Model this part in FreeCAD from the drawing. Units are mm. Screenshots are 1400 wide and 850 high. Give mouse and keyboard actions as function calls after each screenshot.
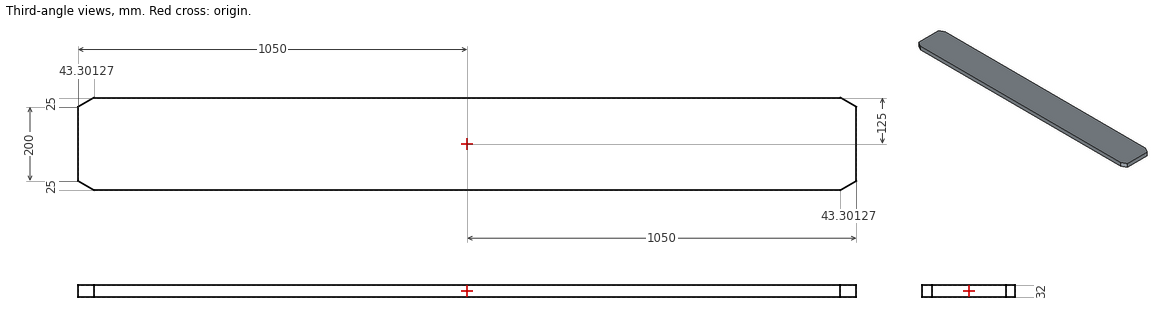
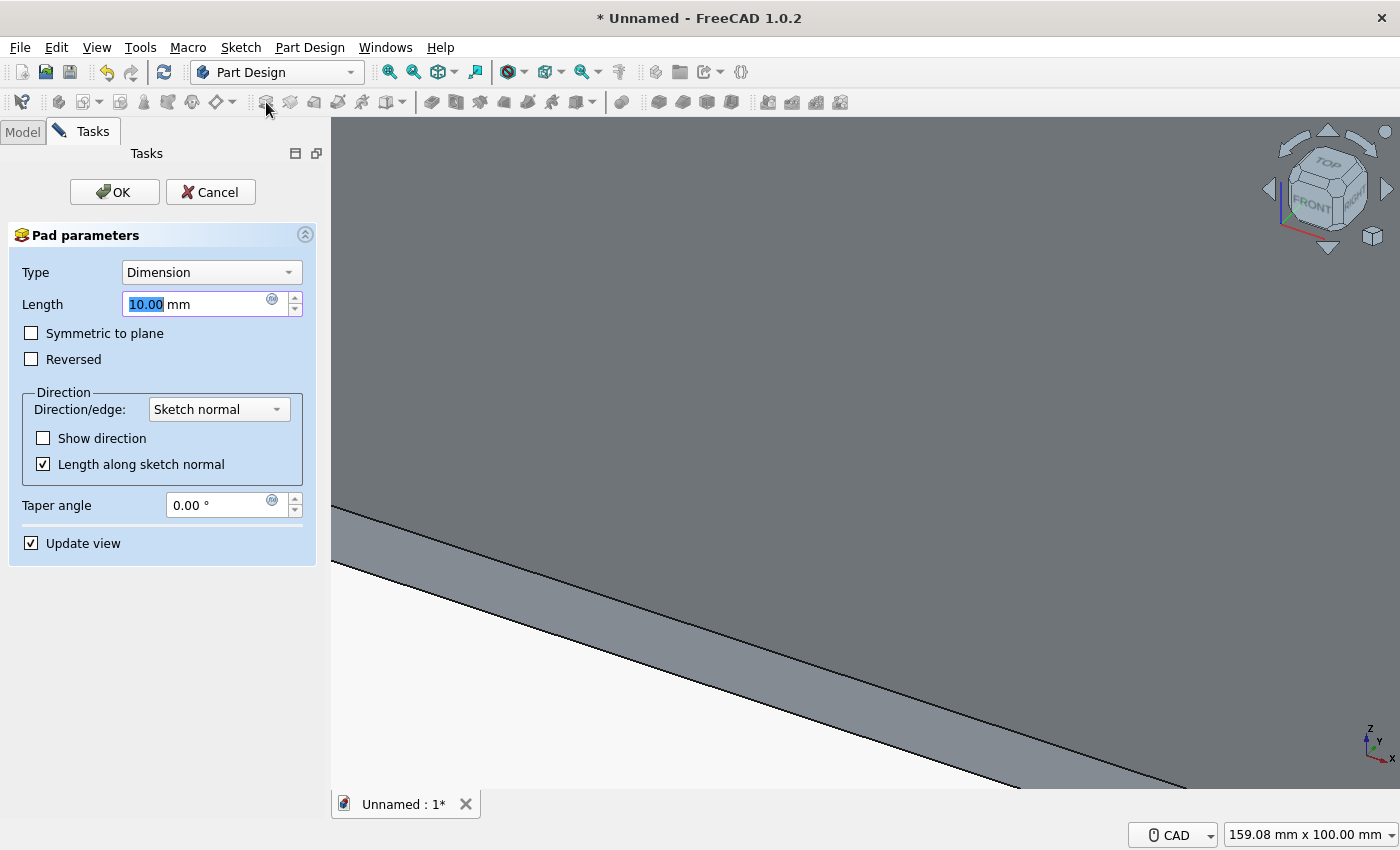
text(32)
key(Tab)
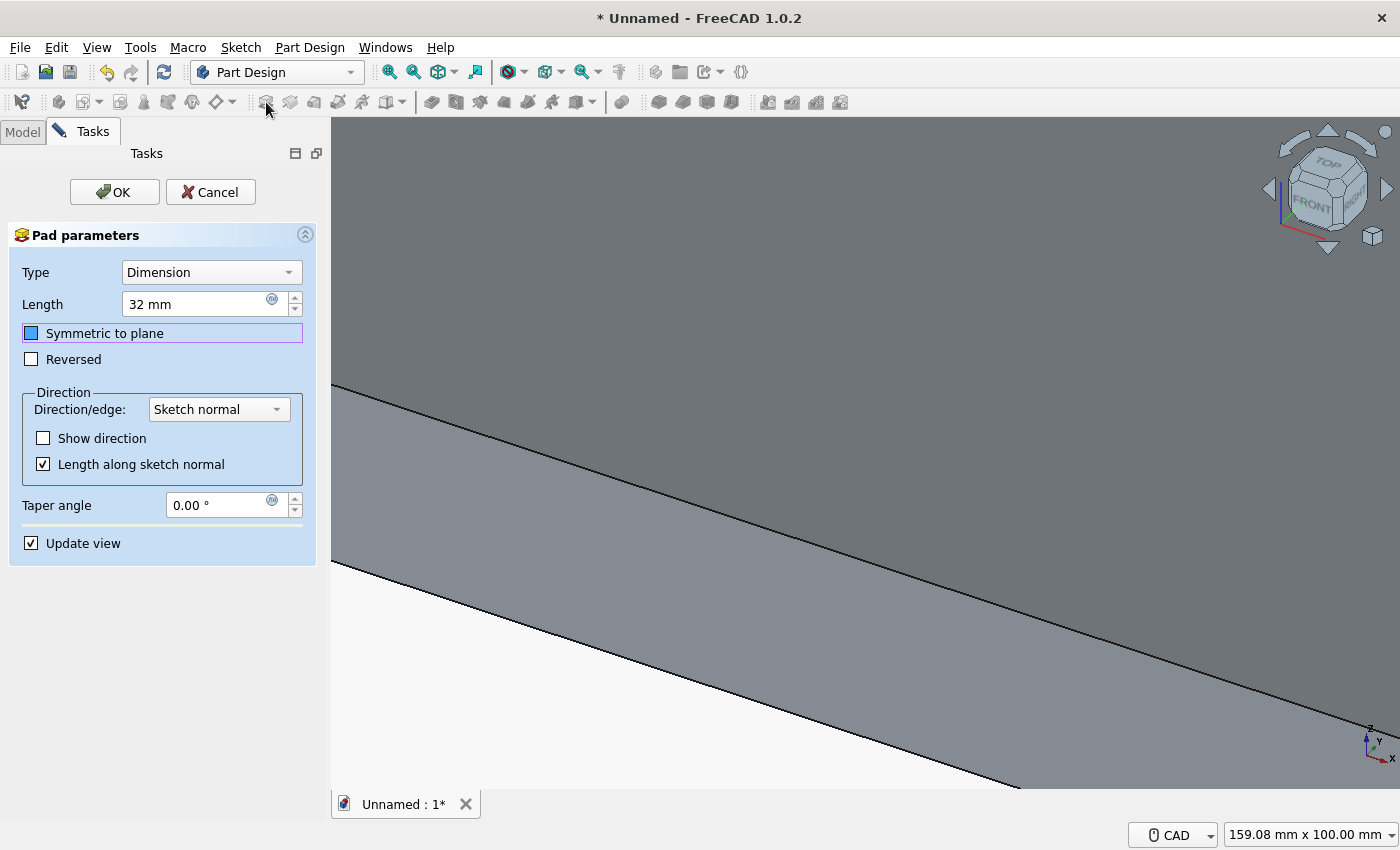
click(30, 333)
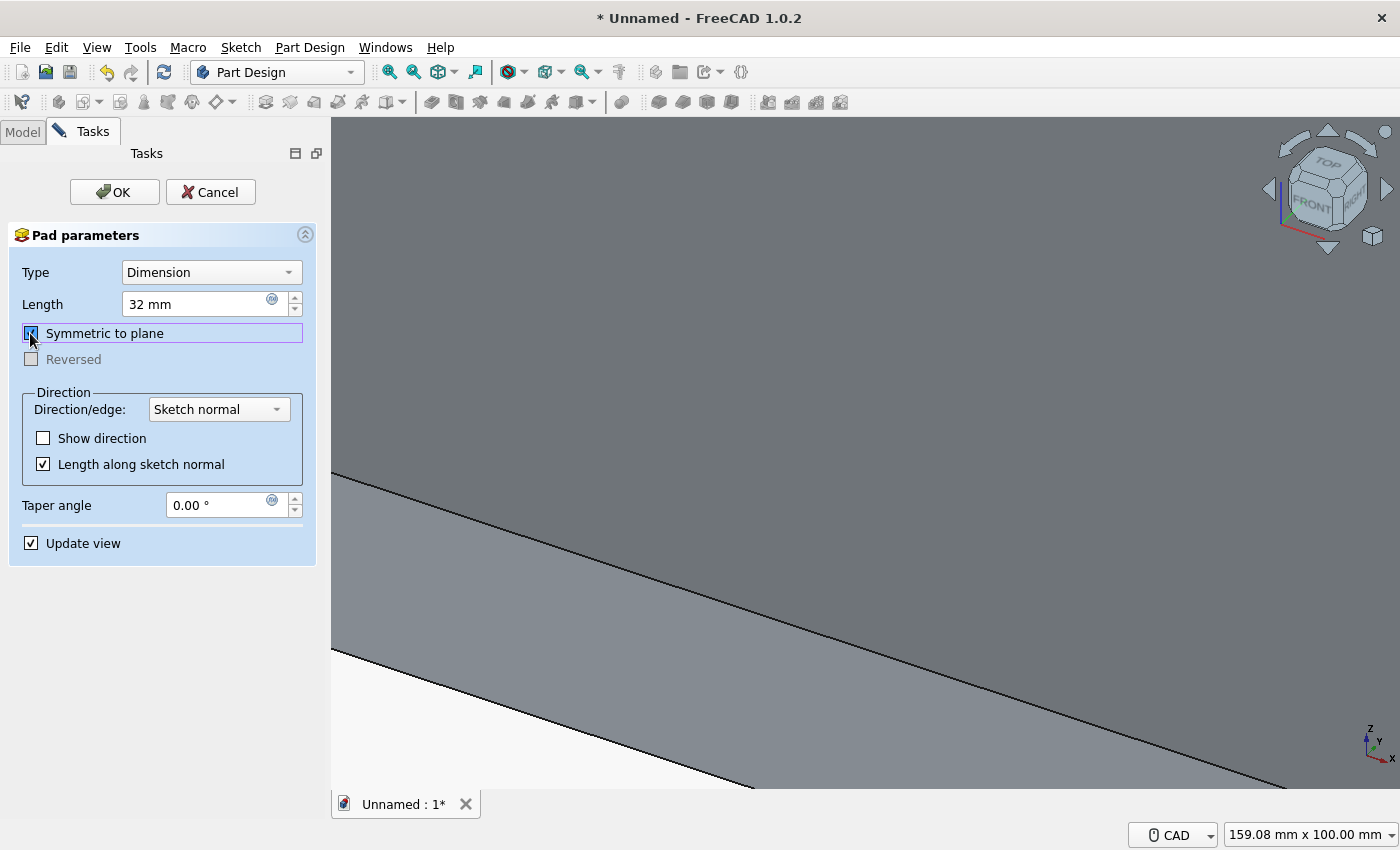
click(115, 192)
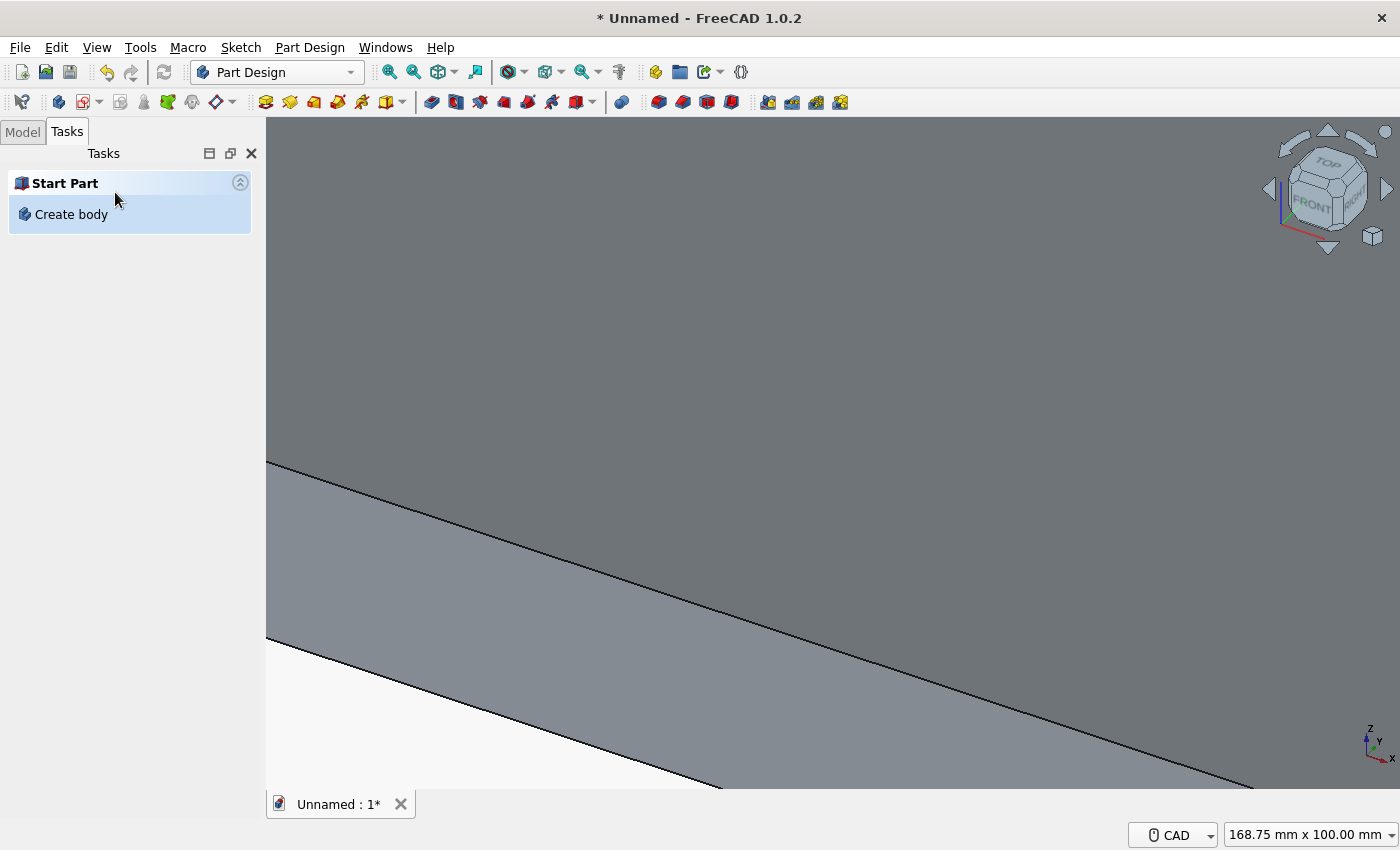
key(0)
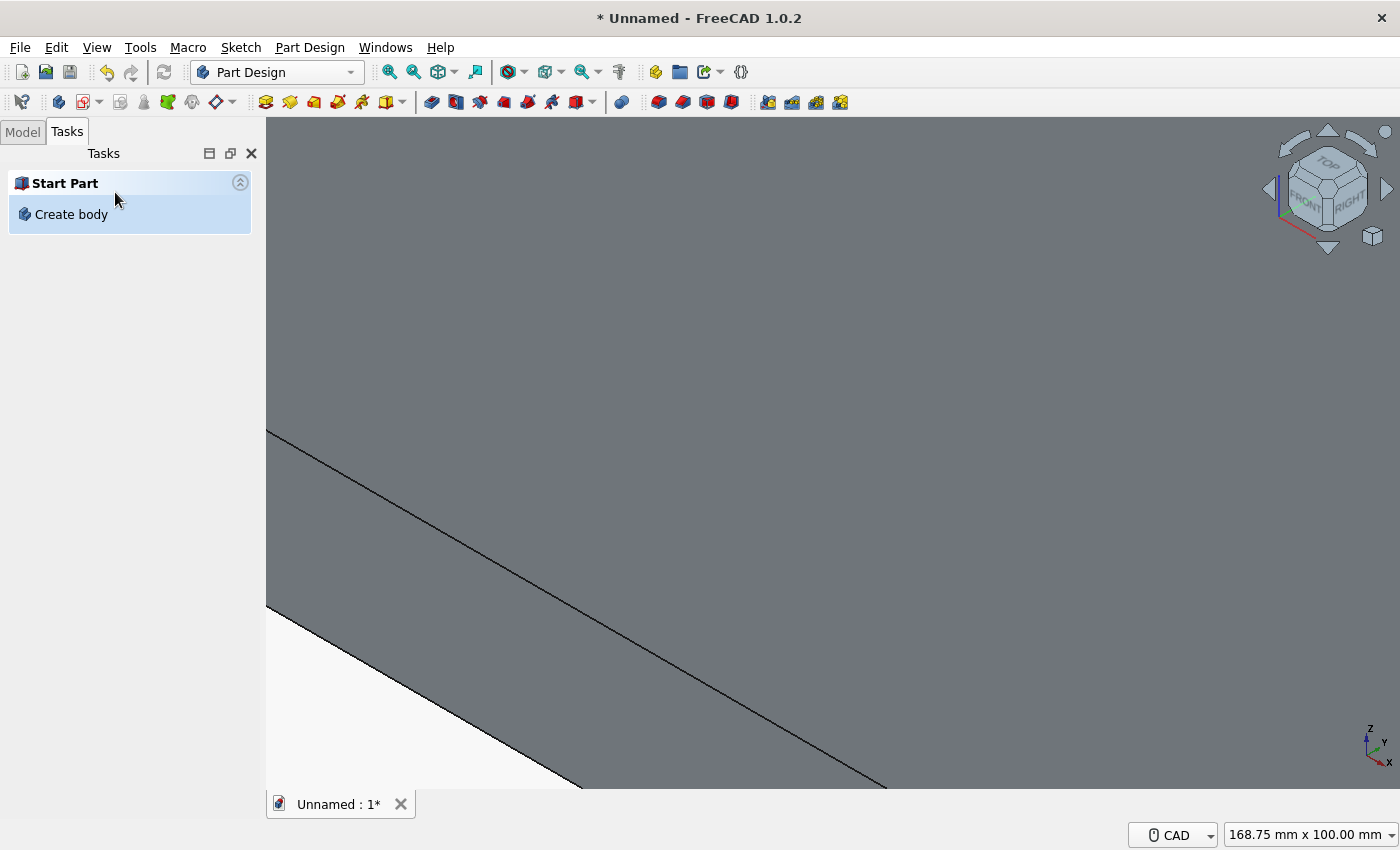
key(v)
key(f)